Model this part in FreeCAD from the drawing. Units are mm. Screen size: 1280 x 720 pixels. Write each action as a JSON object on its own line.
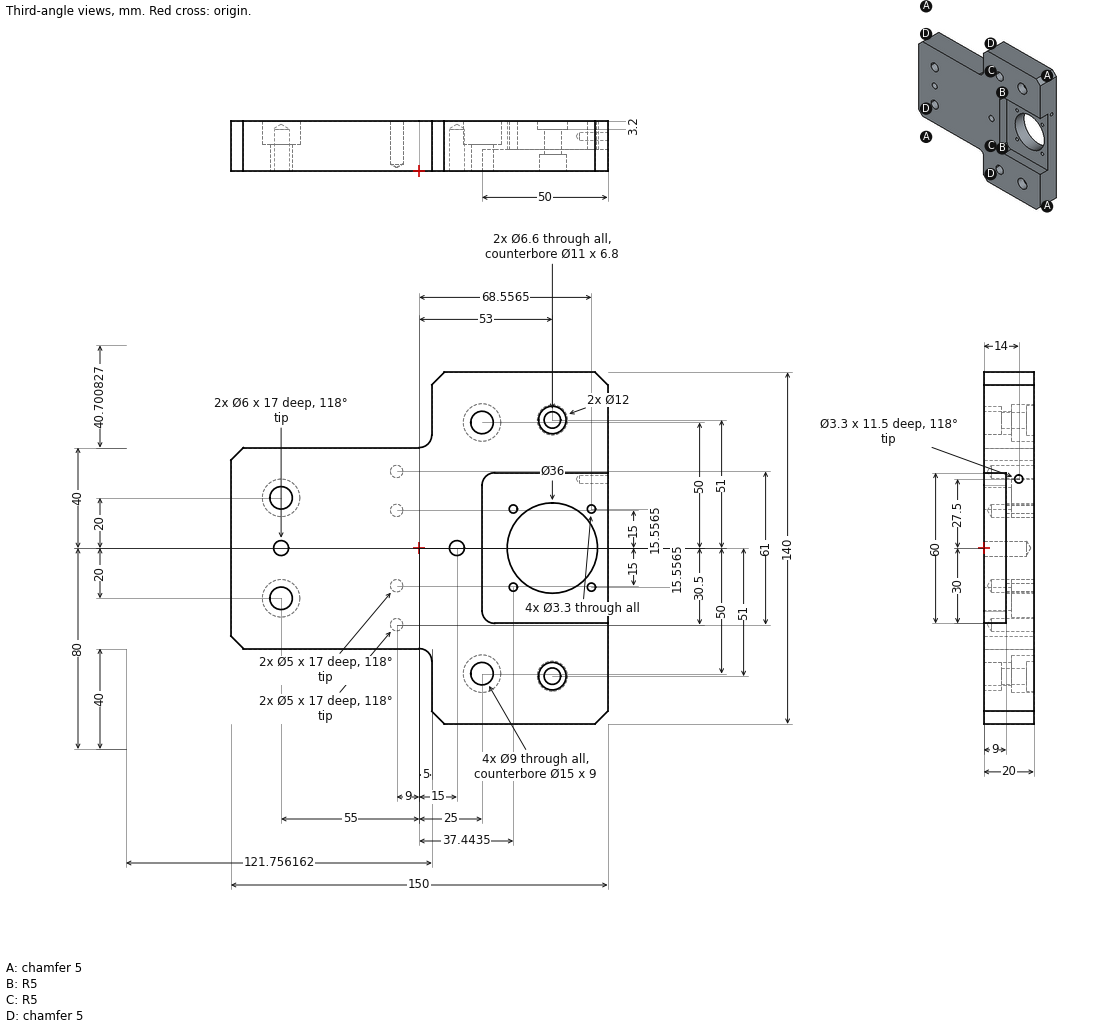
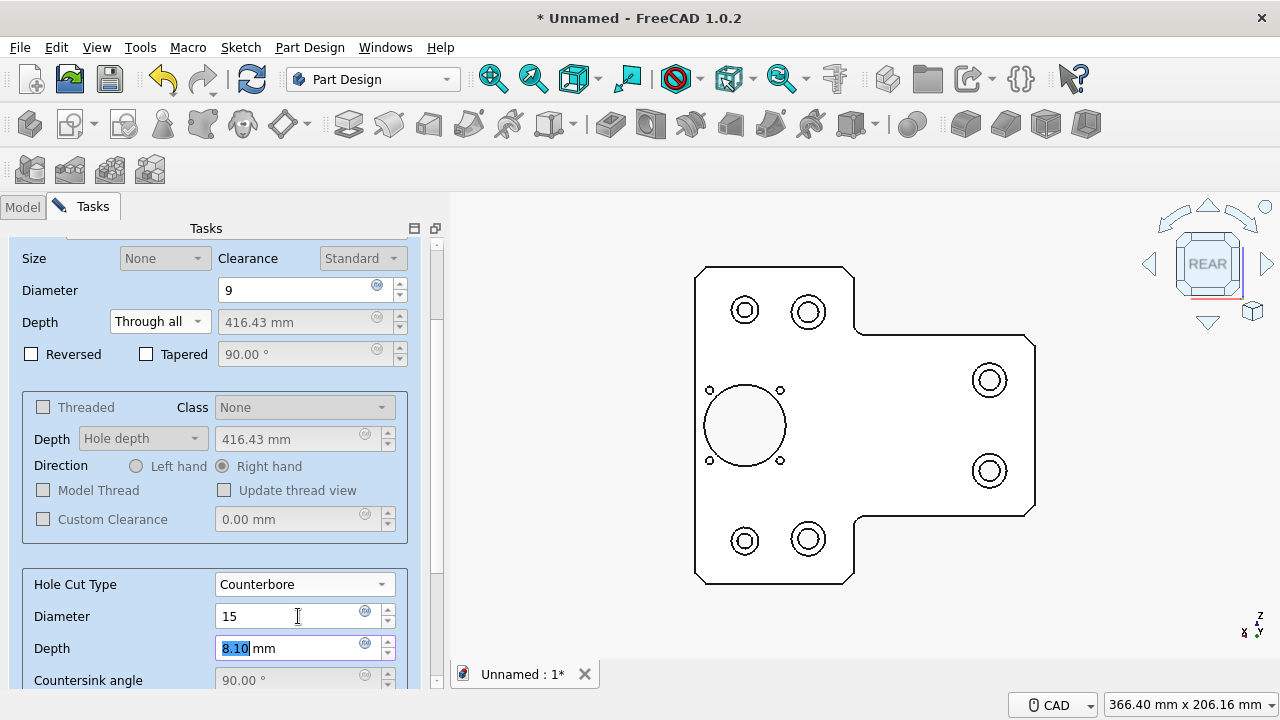
{"action": "type", "text": "9"}
{"action": "key", "text": "Tab"}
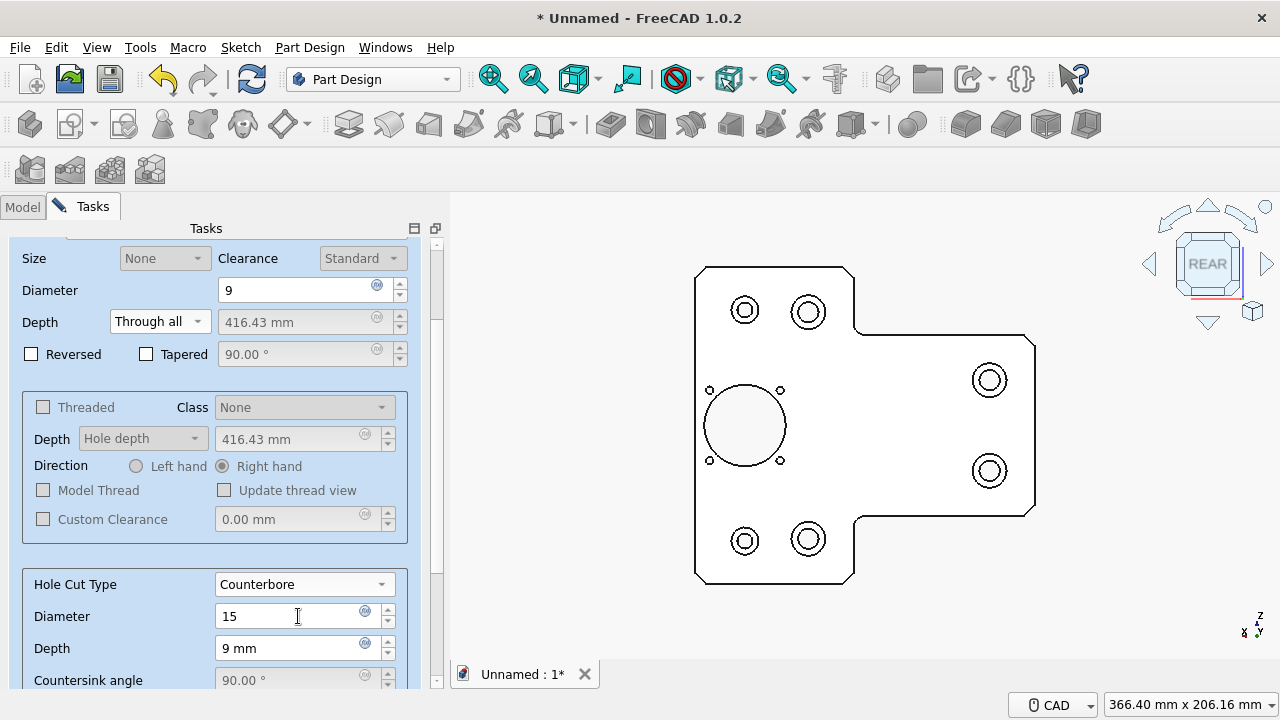
{"action": "scroll", "coordinate": [437, 463], "scroll_direction": "up", "scroll_amount": 3}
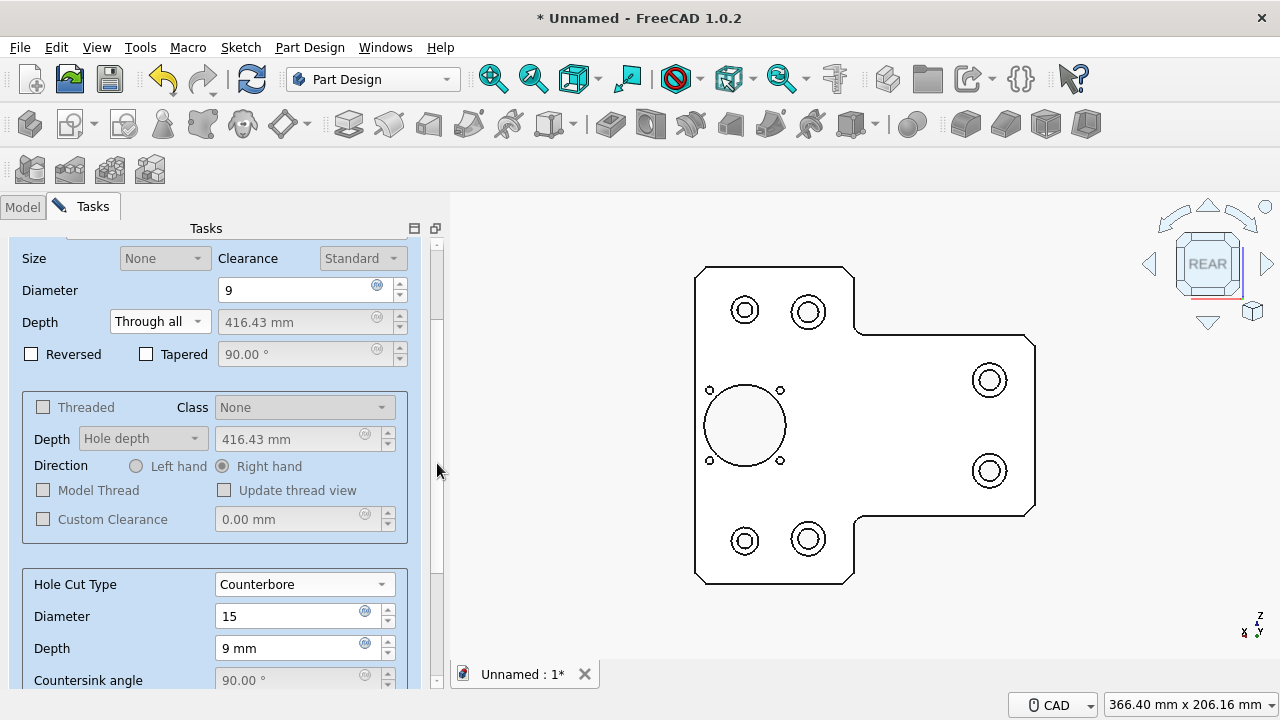
{"action": "left_click", "coordinate": [167, 267]}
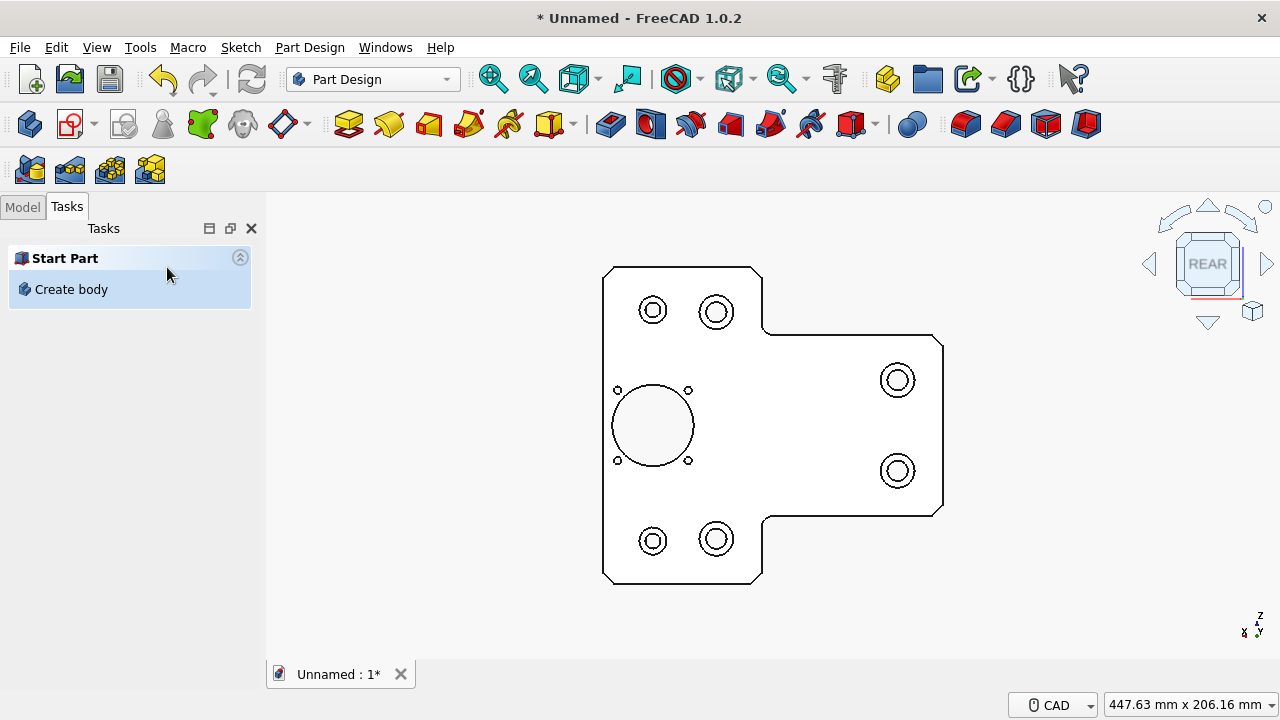
{"action": "left_click", "coordinate": [773, 424]}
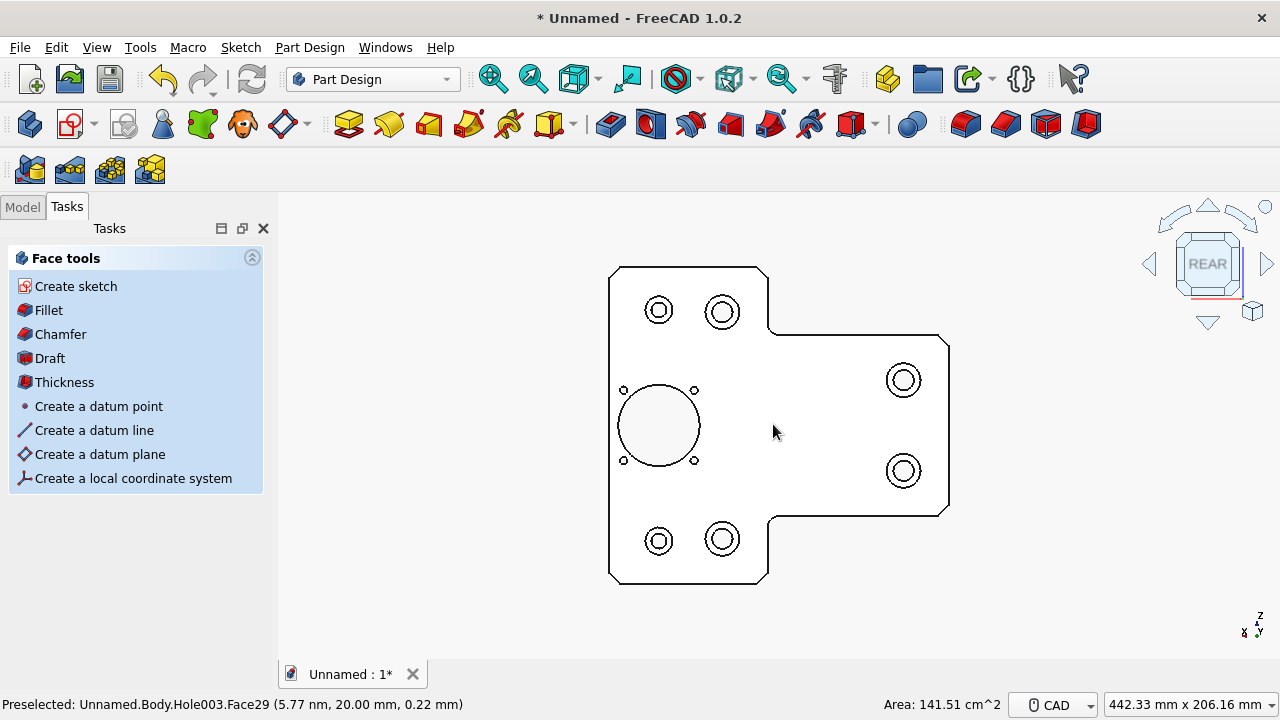
{"action": "left_click", "coordinate": [70, 124]}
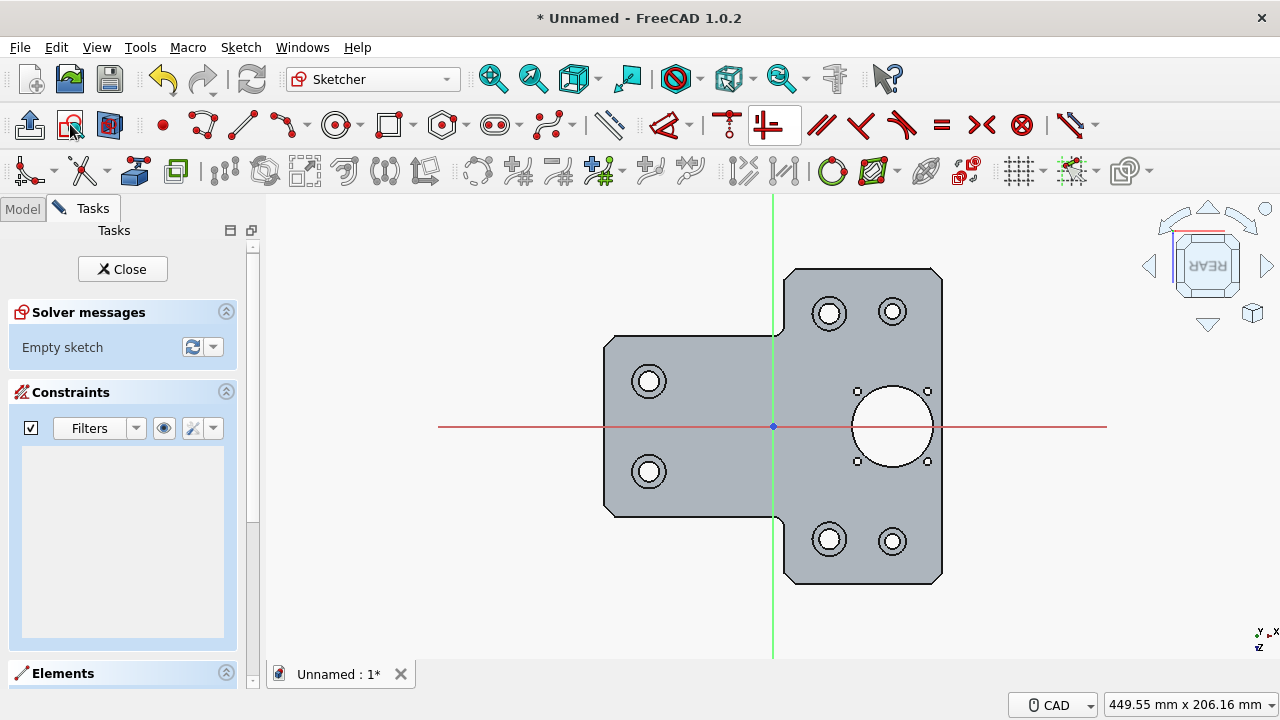
{"action": "scroll", "coordinate": [828, 426], "scroll_direction": "up", "scroll_amount": 3}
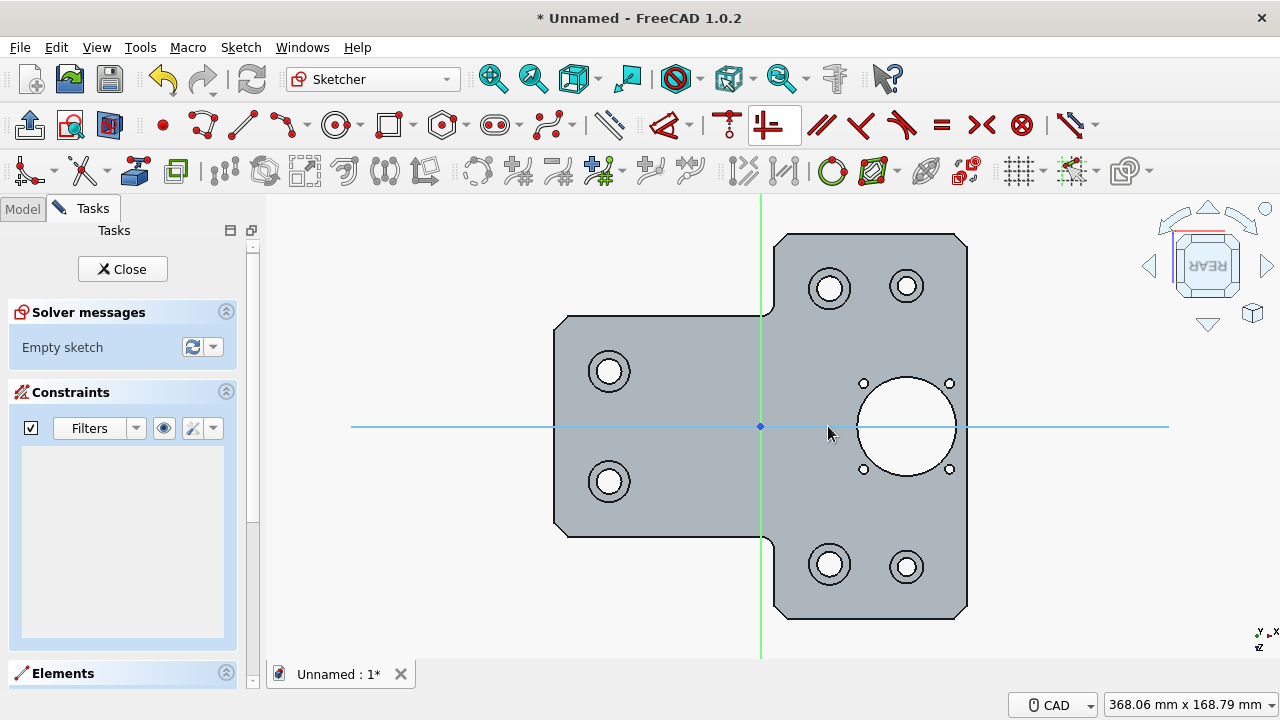
{"action": "left_click", "coordinate": [336, 126]}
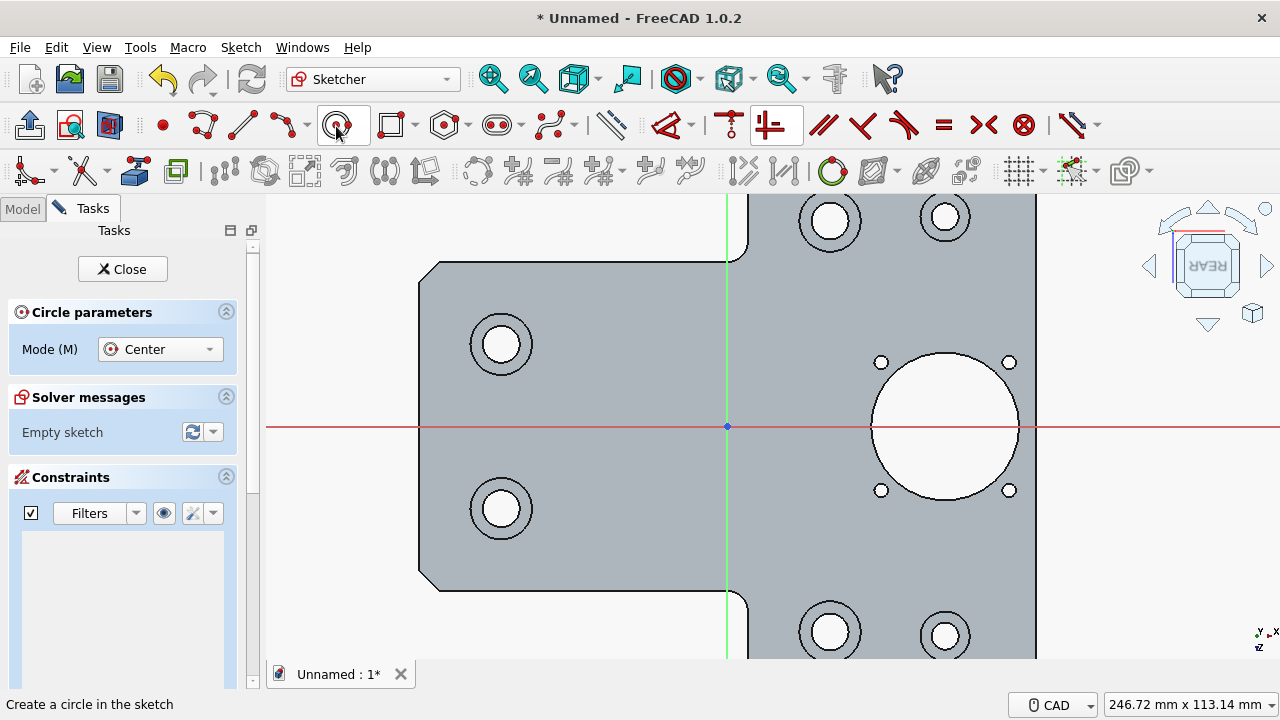
{"action": "scroll", "coordinate": [690, 301], "scroll_direction": "up", "scroll_amount": 4}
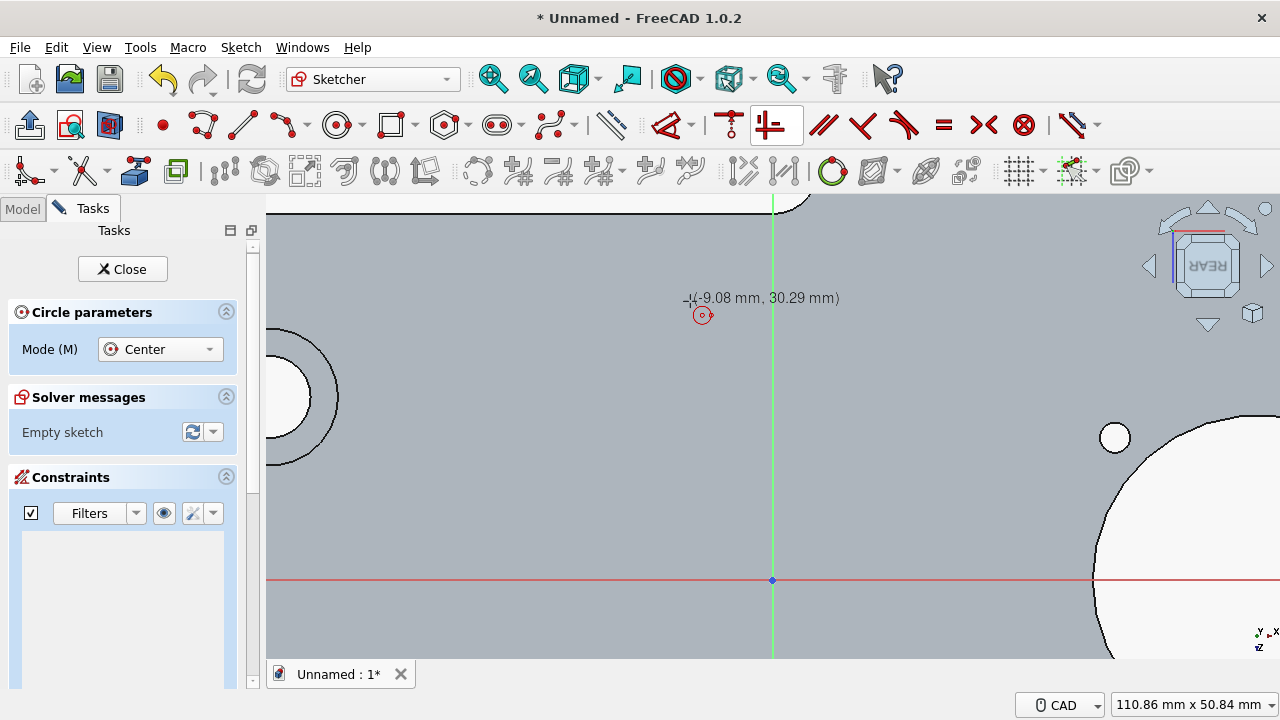
{"action": "left_click", "coordinate": [690, 301]}
{"action": "left_click", "coordinate": [706, 285]}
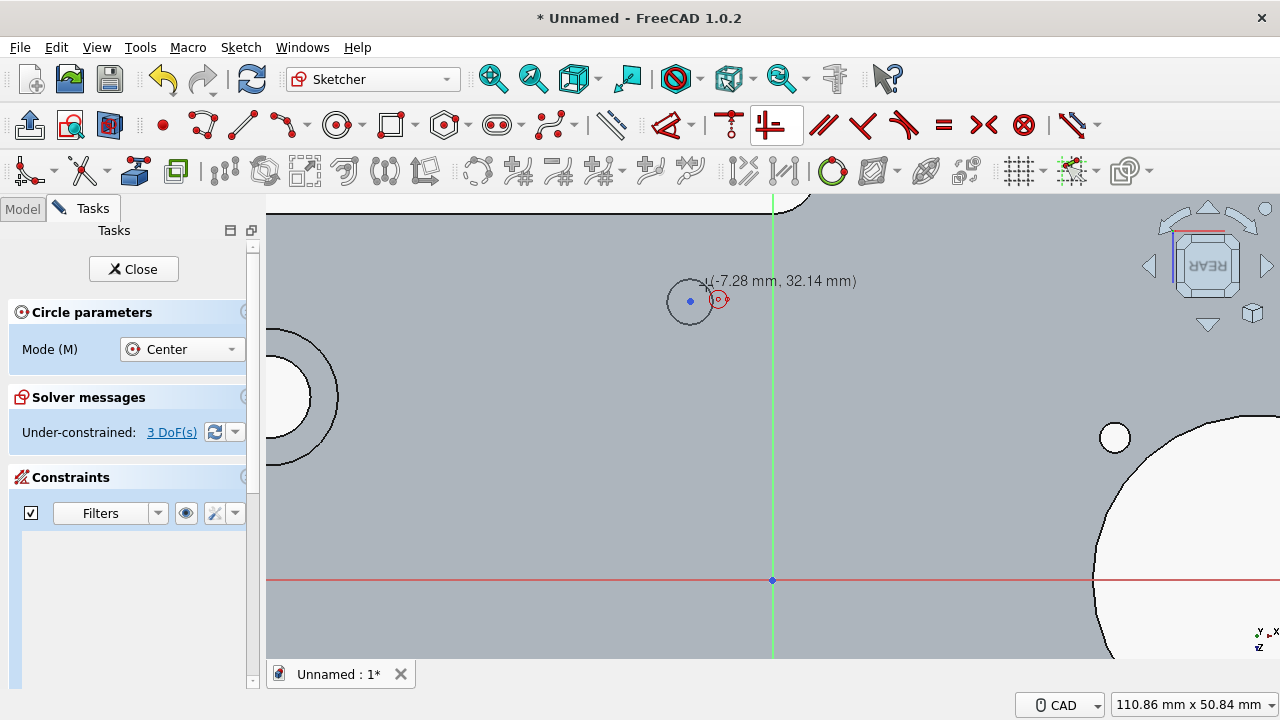
{"action": "scroll", "coordinate": [692, 301], "scroll_direction": "down", "scroll_amount": 4}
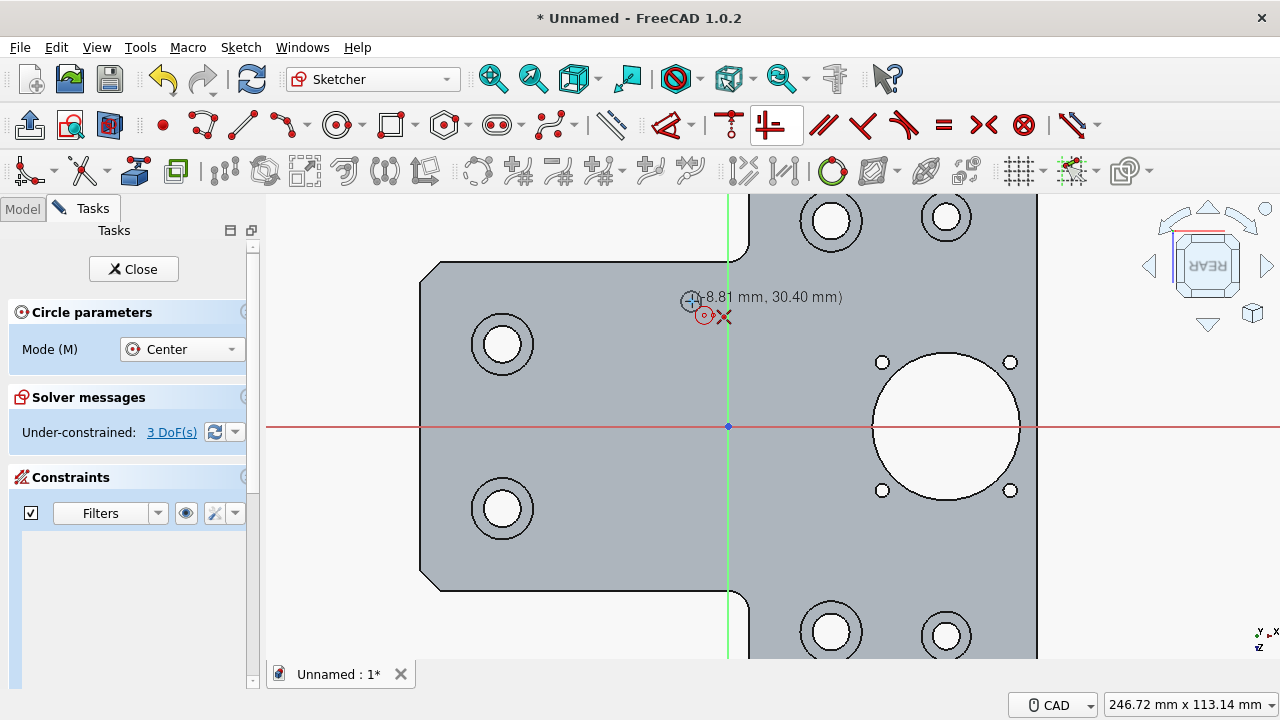
{"action": "scroll", "coordinate": [691, 552], "scroll_direction": "up", "scroll_amount": 4}